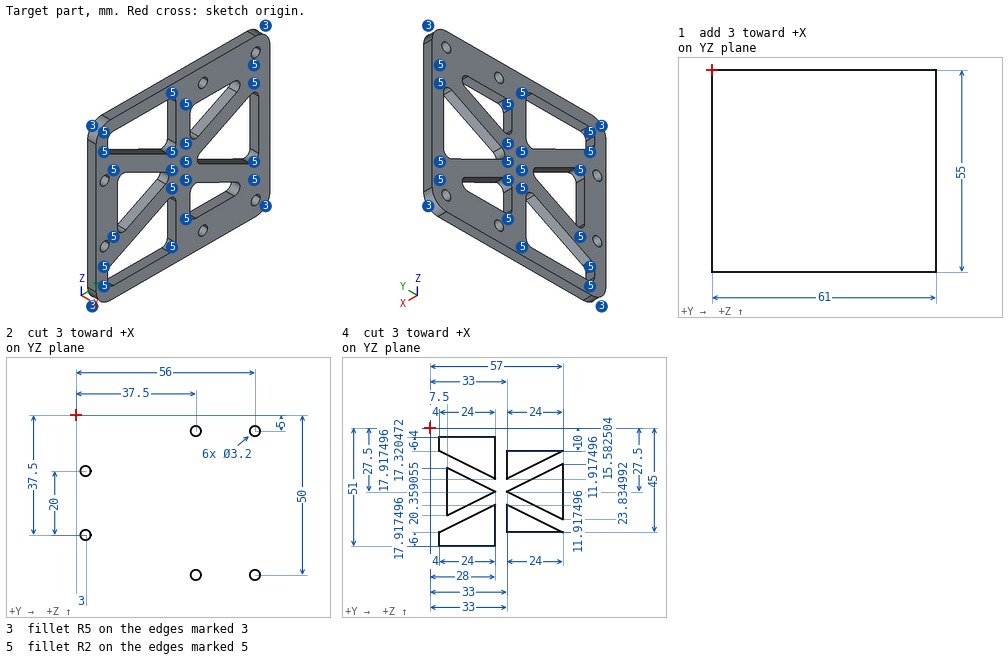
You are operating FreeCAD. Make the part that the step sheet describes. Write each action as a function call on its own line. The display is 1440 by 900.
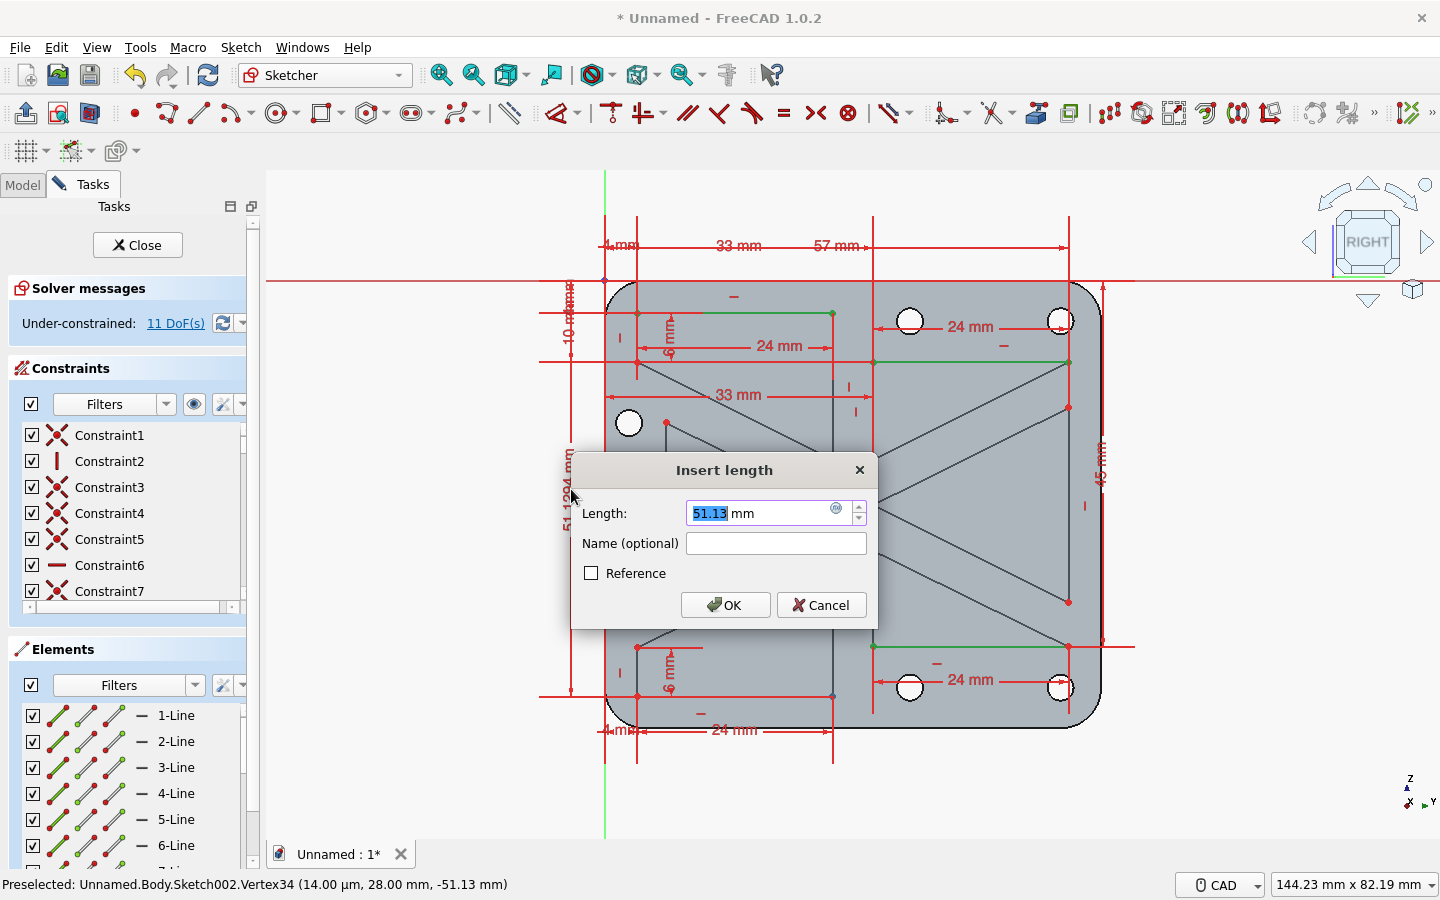
text(51)
key(Return)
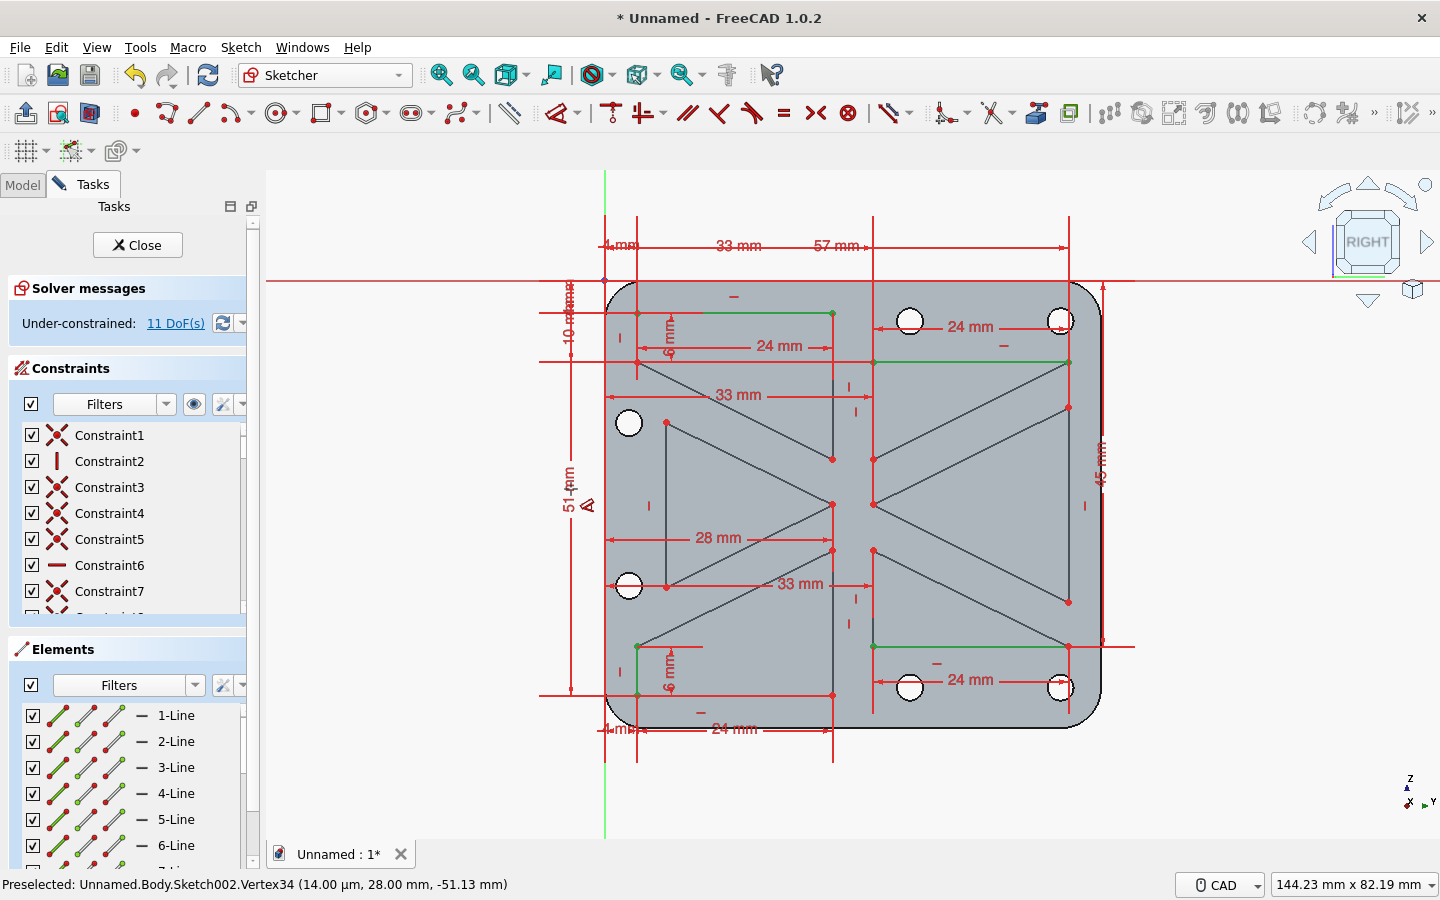
click(666, 423)
click(635, 457)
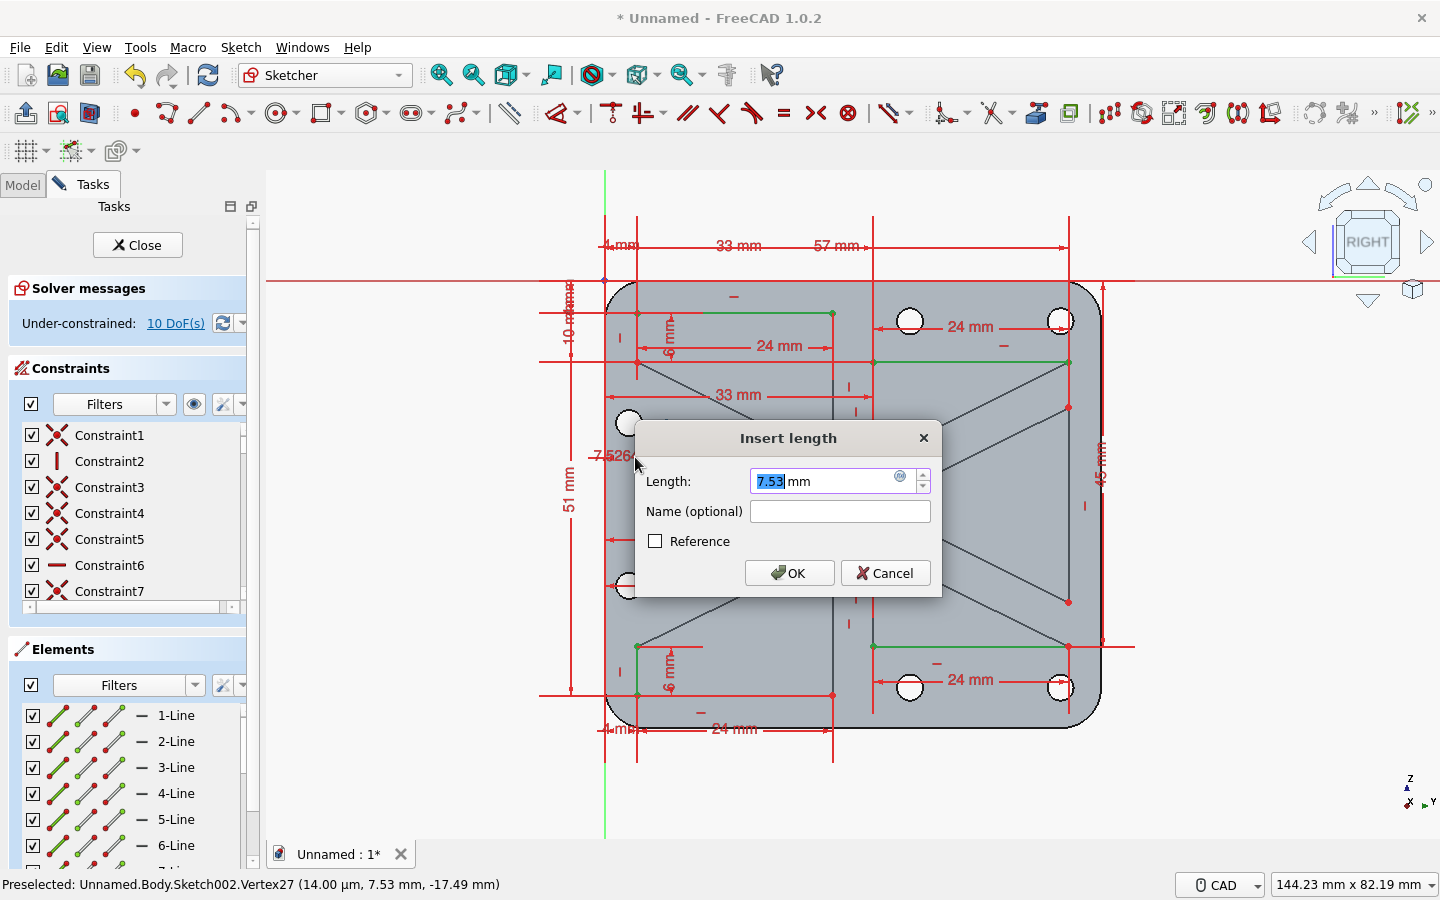
text(7.5)
key(Return)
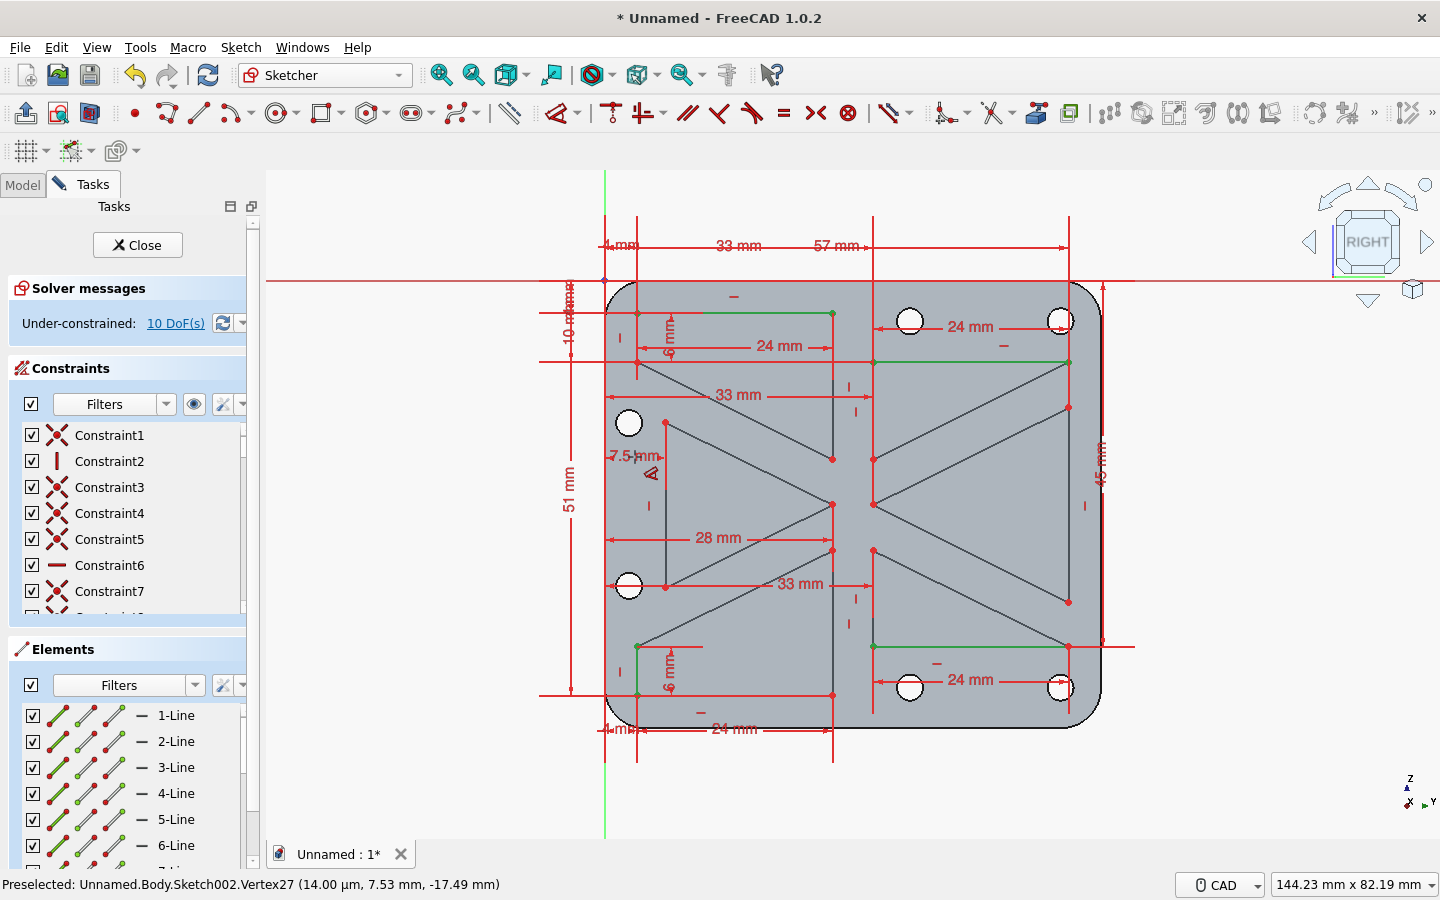
click(873, 505)
click(571, 393)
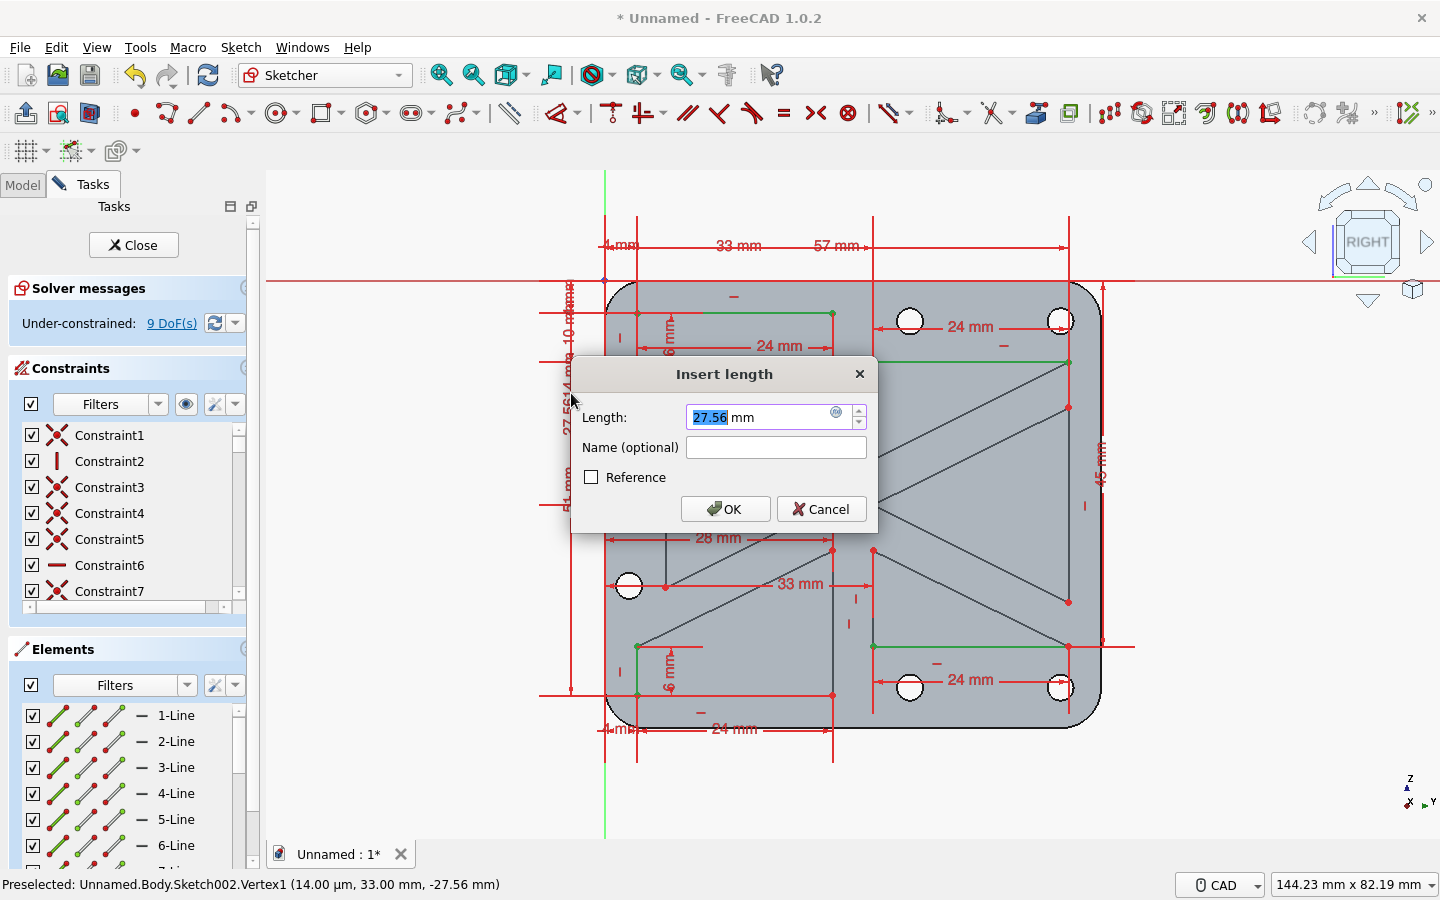
text(27.5)
key(Return)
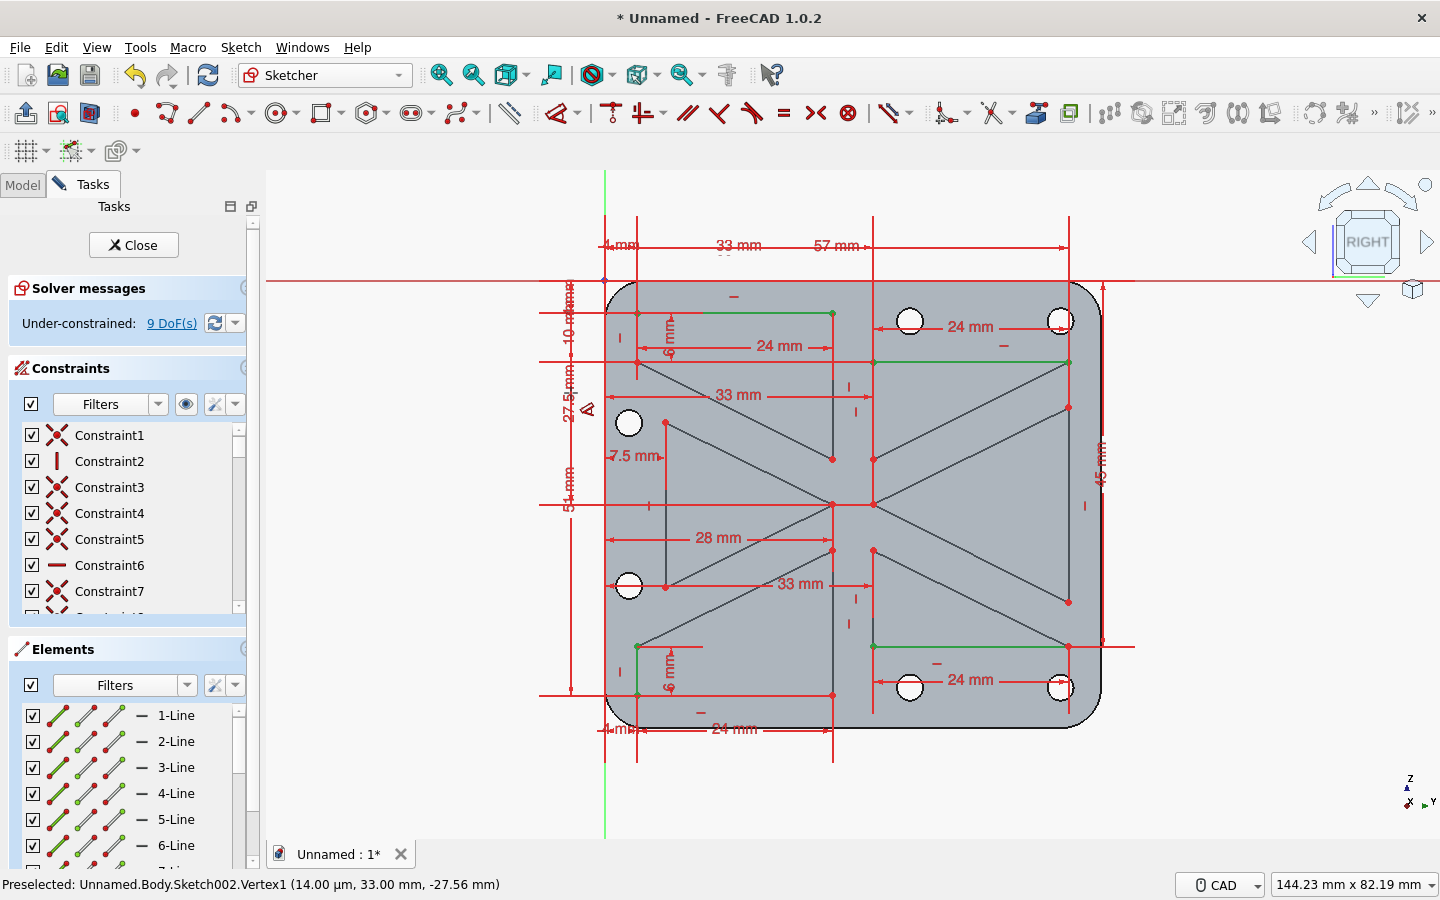
click(833, 505)
click(867, 341)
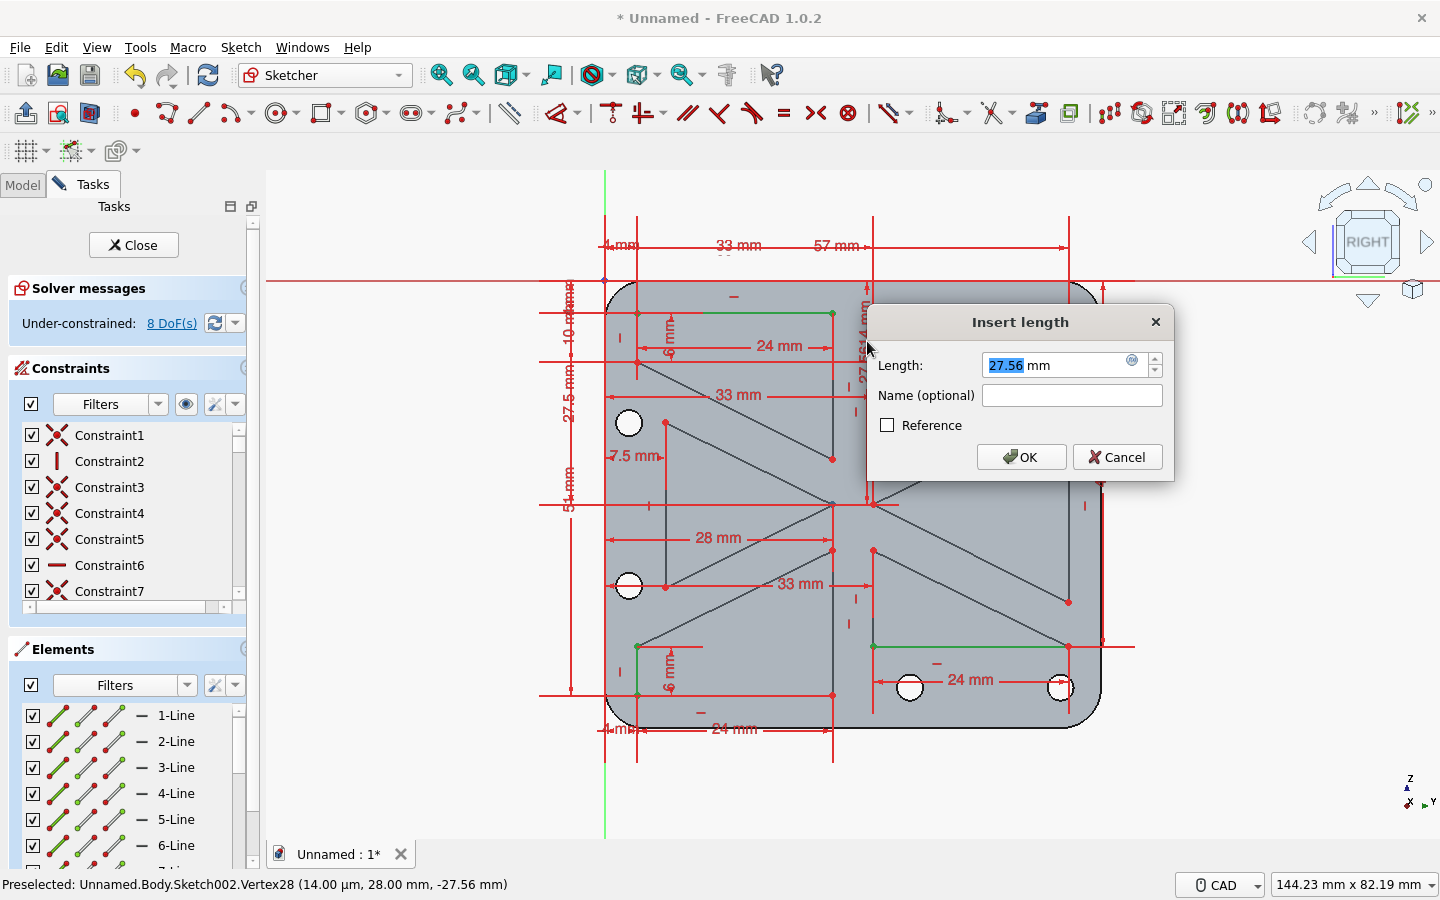
text(27.5)
key(Return)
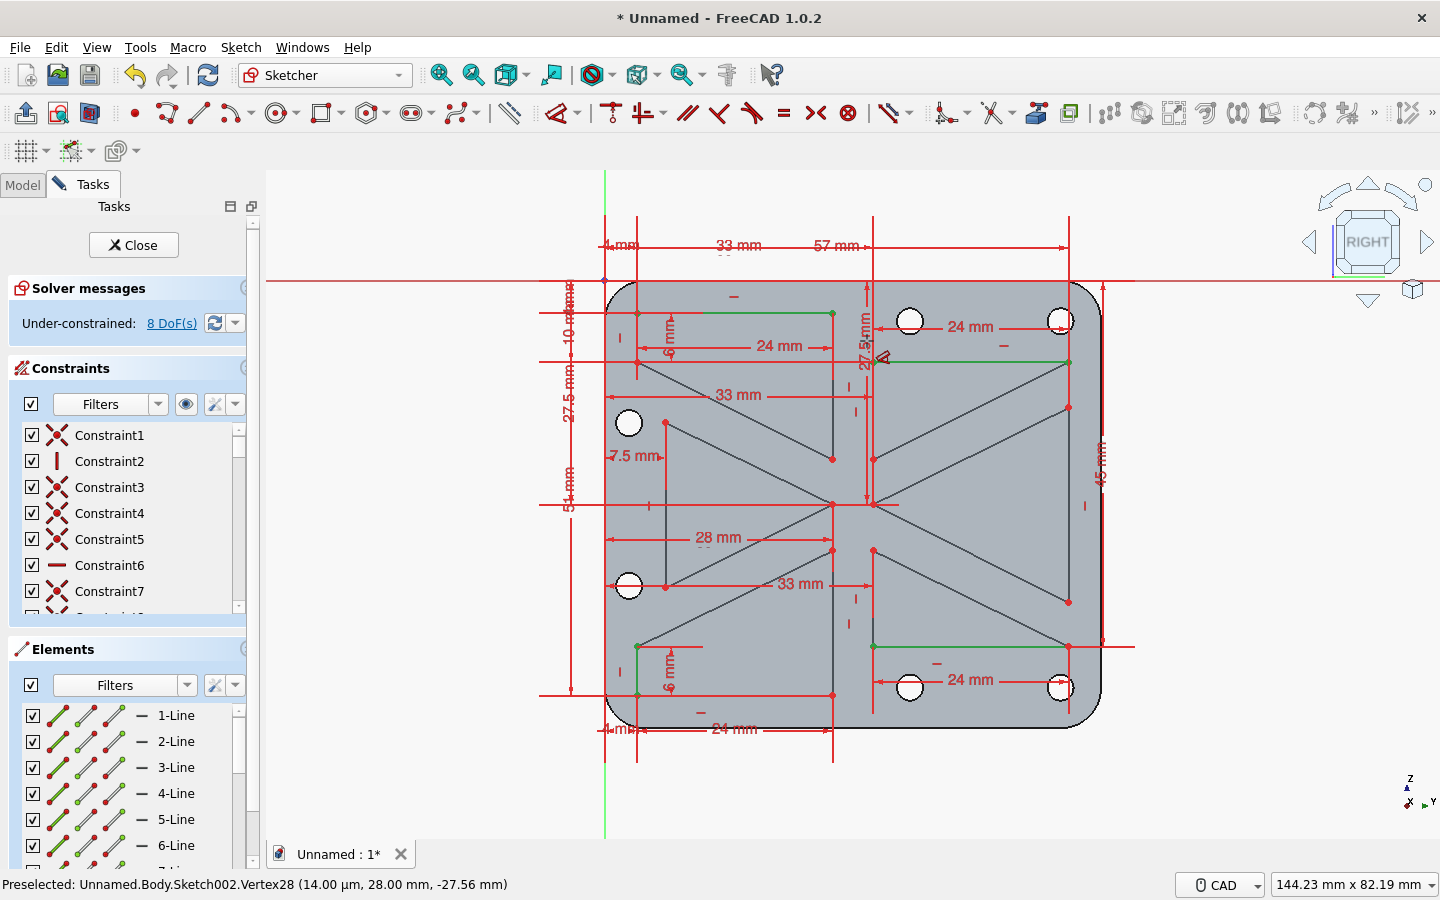
click(1069, 467)
click(1103, 506)